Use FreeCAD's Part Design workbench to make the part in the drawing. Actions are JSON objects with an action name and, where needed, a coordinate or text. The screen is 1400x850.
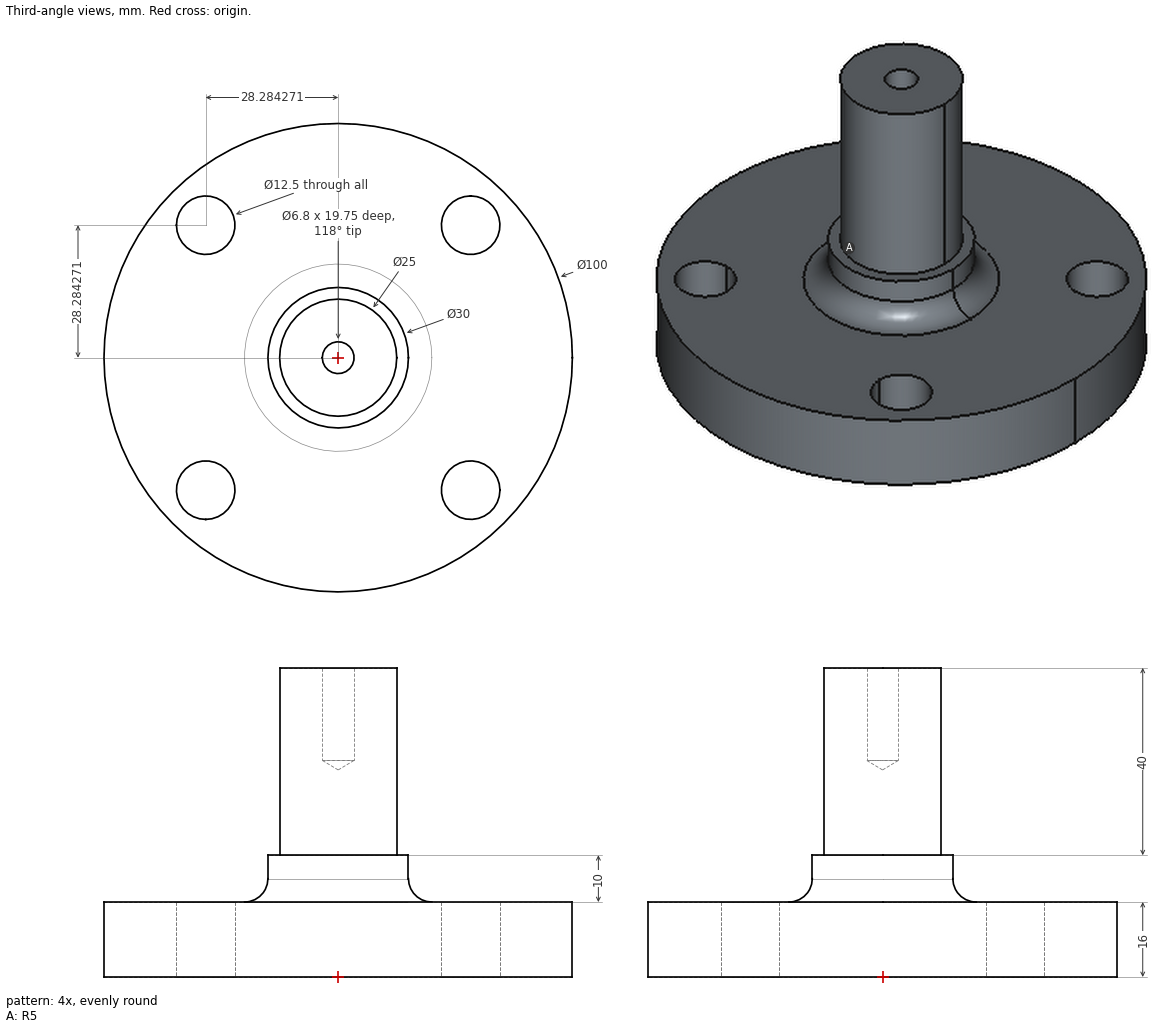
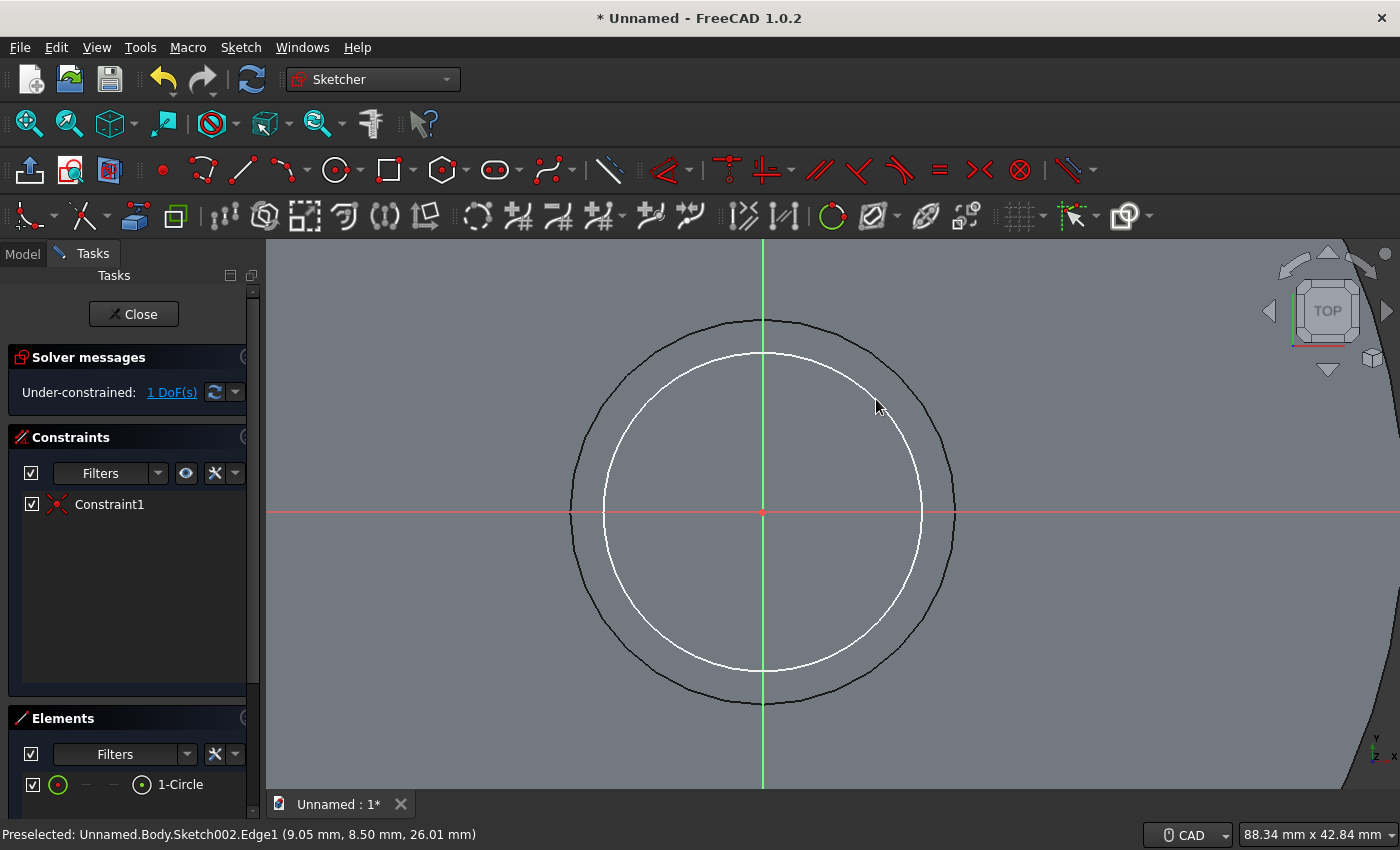
{"action": "left_click", "coordinate": [664, 170]}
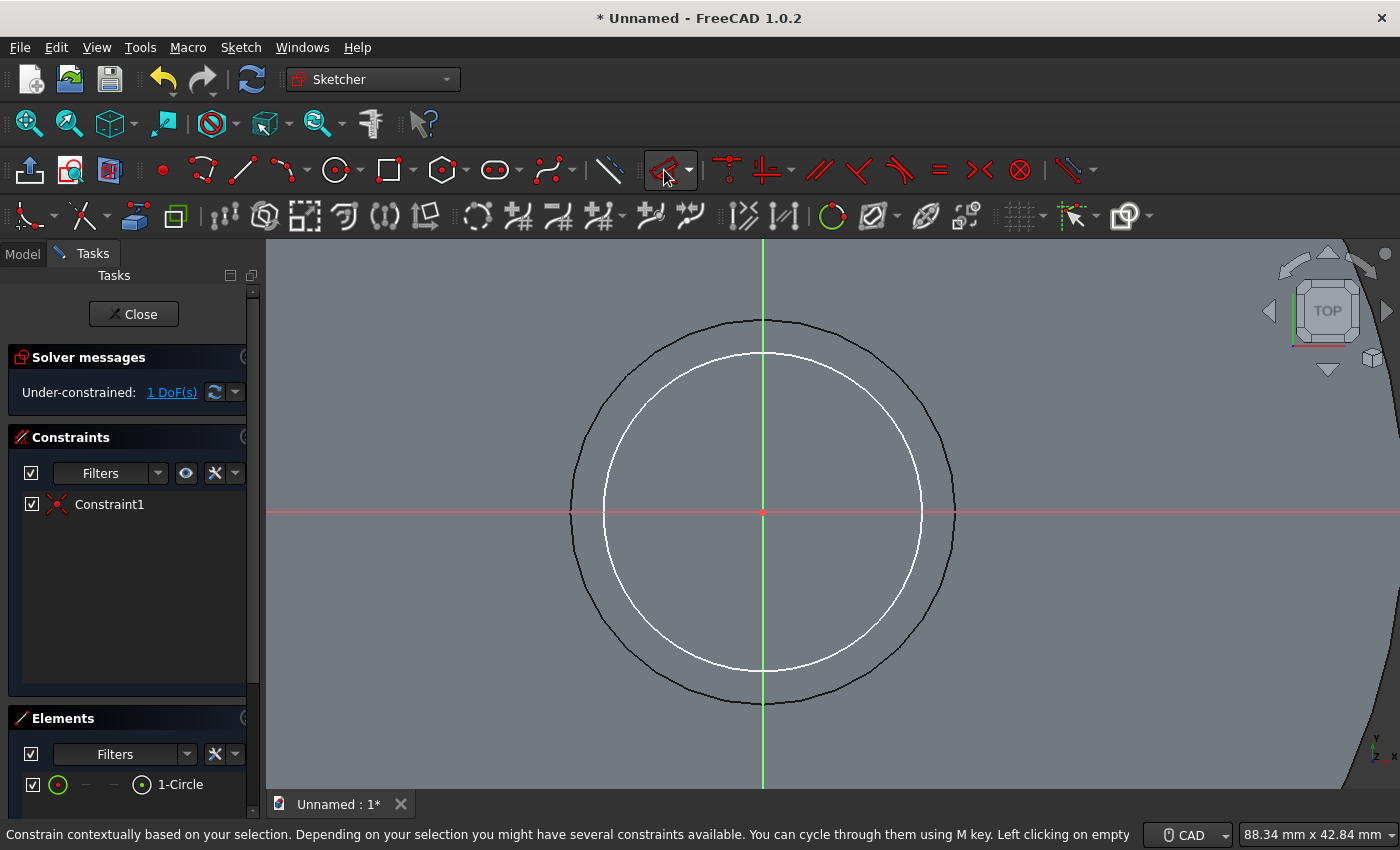
{"action": "left_click", "coordinate": [875, 399]}
{"action": "left_click", "coordinate": [898, 376]}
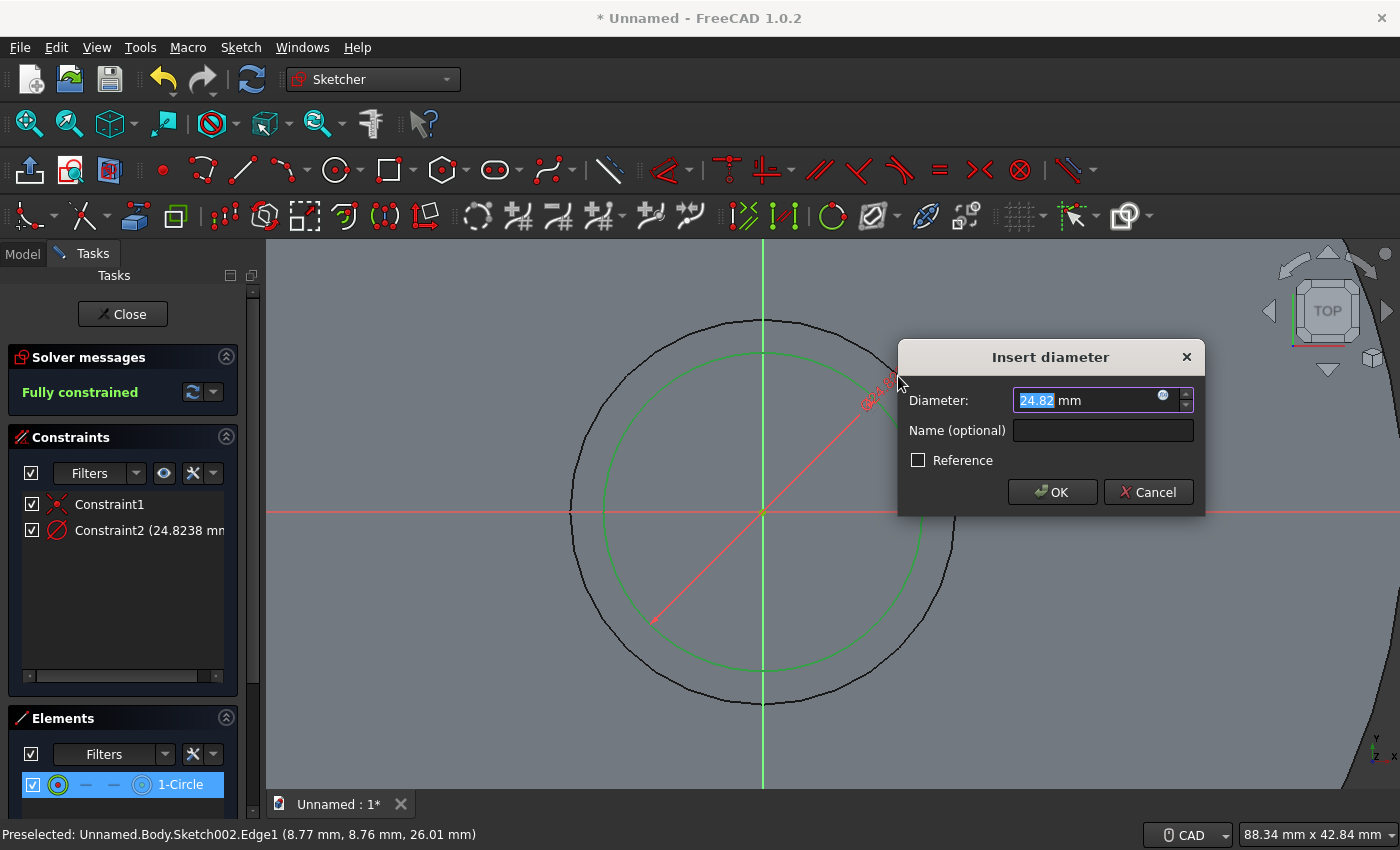
{"action": "type", "text": "25"}
{"action": "key", "text": "Return"}
{"action": "key", "text": "Escape"}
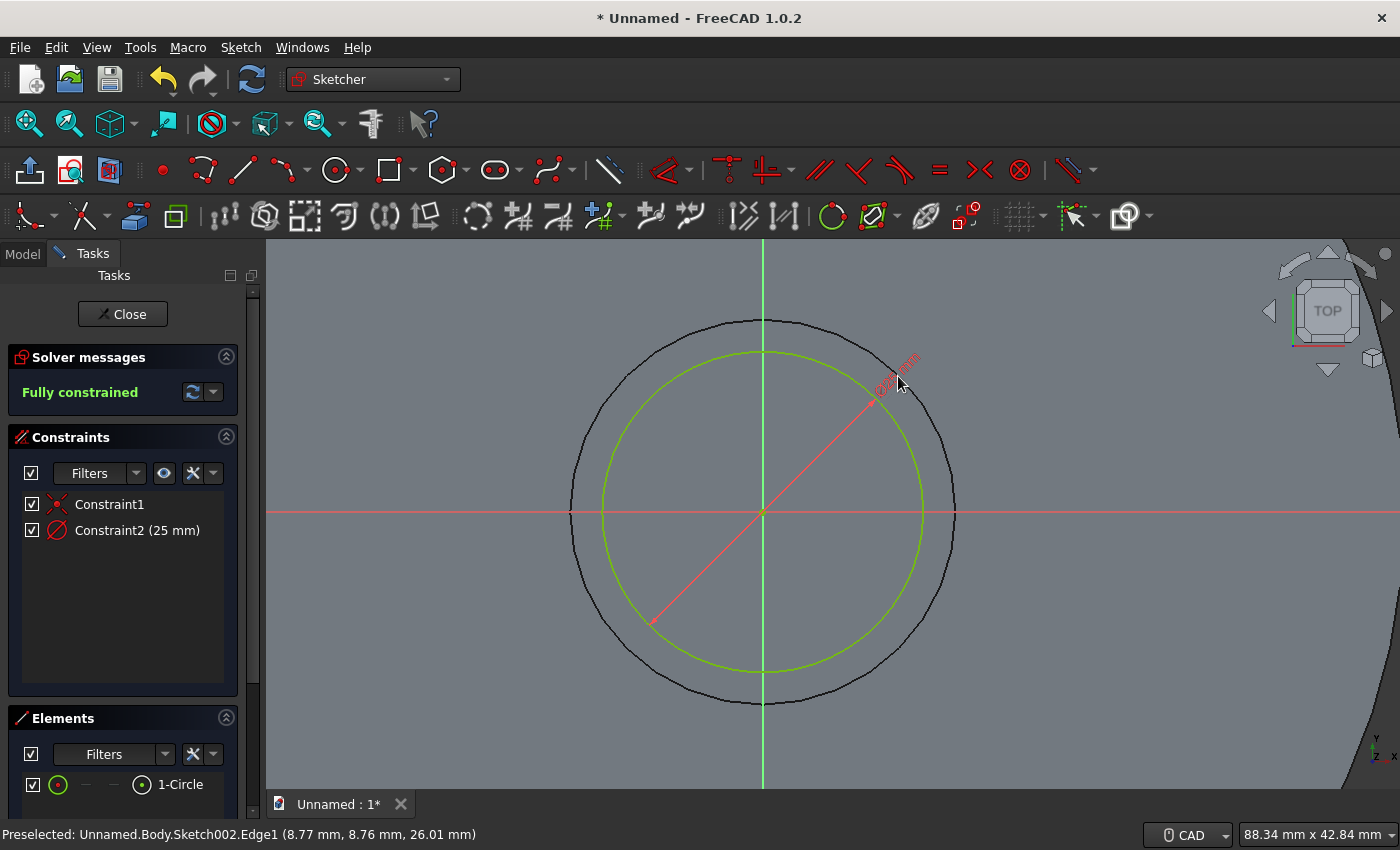
{"action": "left_click", "coordinate": [123, 314]}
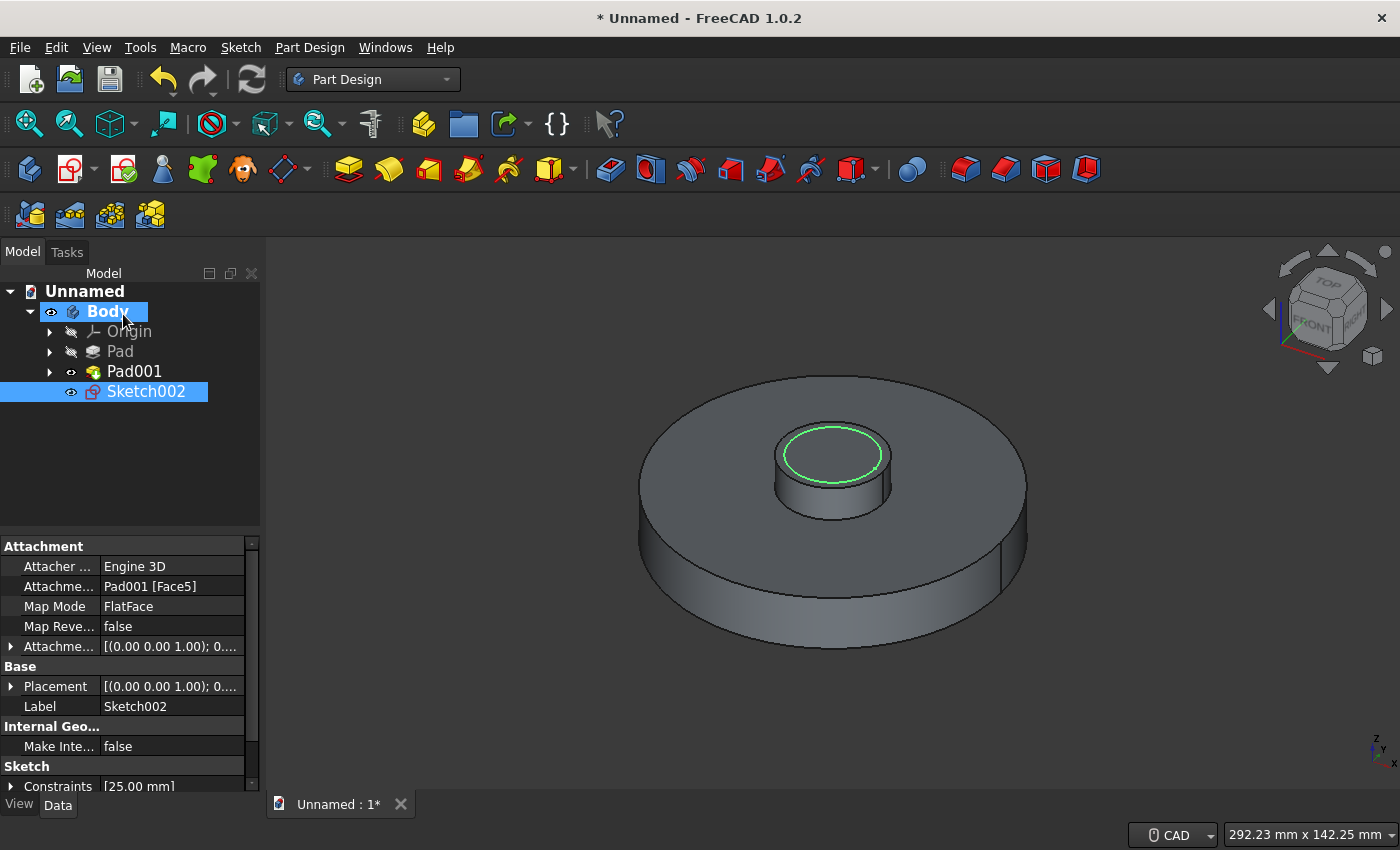
{"action": "left_click", "coordinate": [350, 170]}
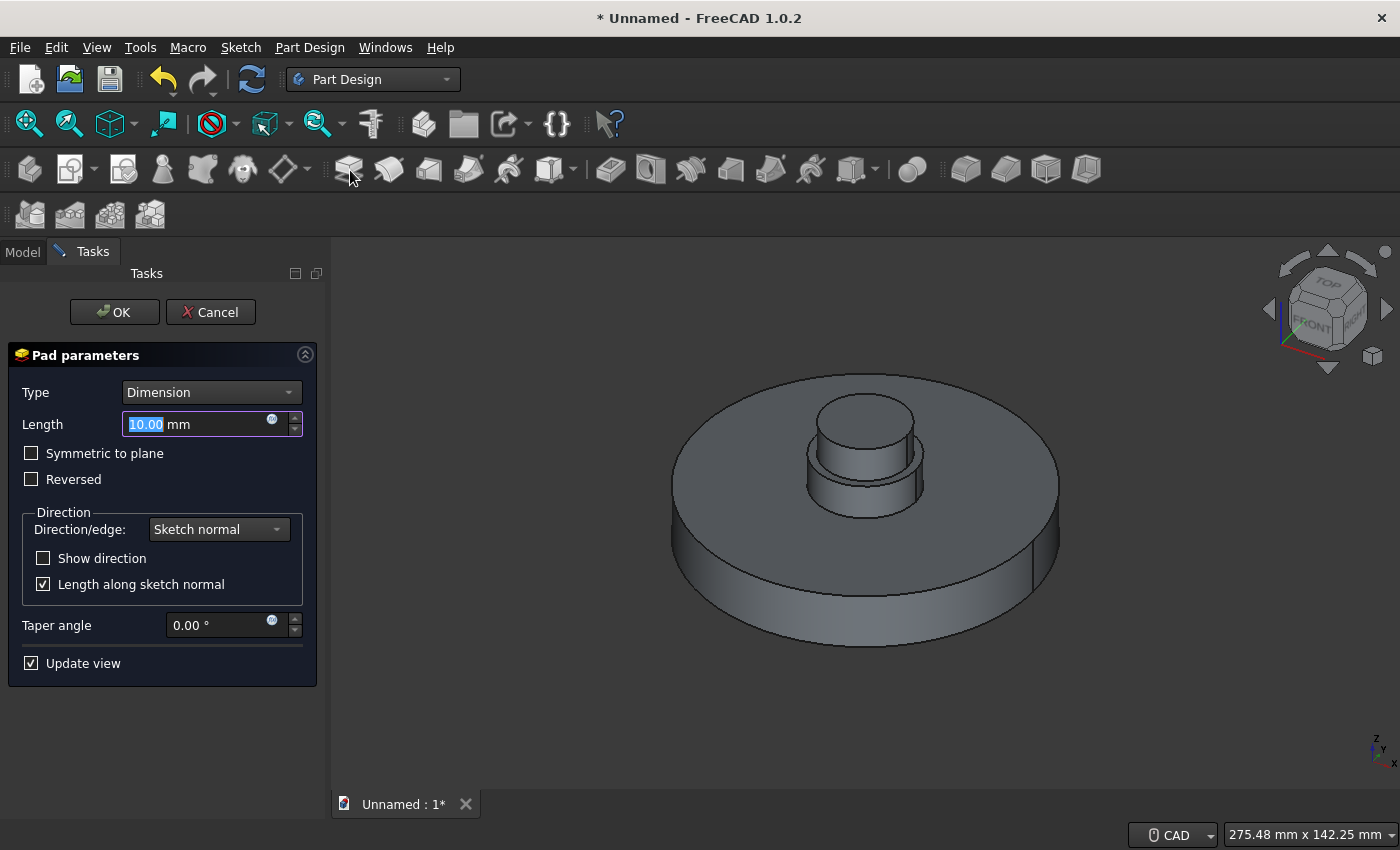
{"action": "type", "text": "40"}
{"action": "key", "text": "Tab"}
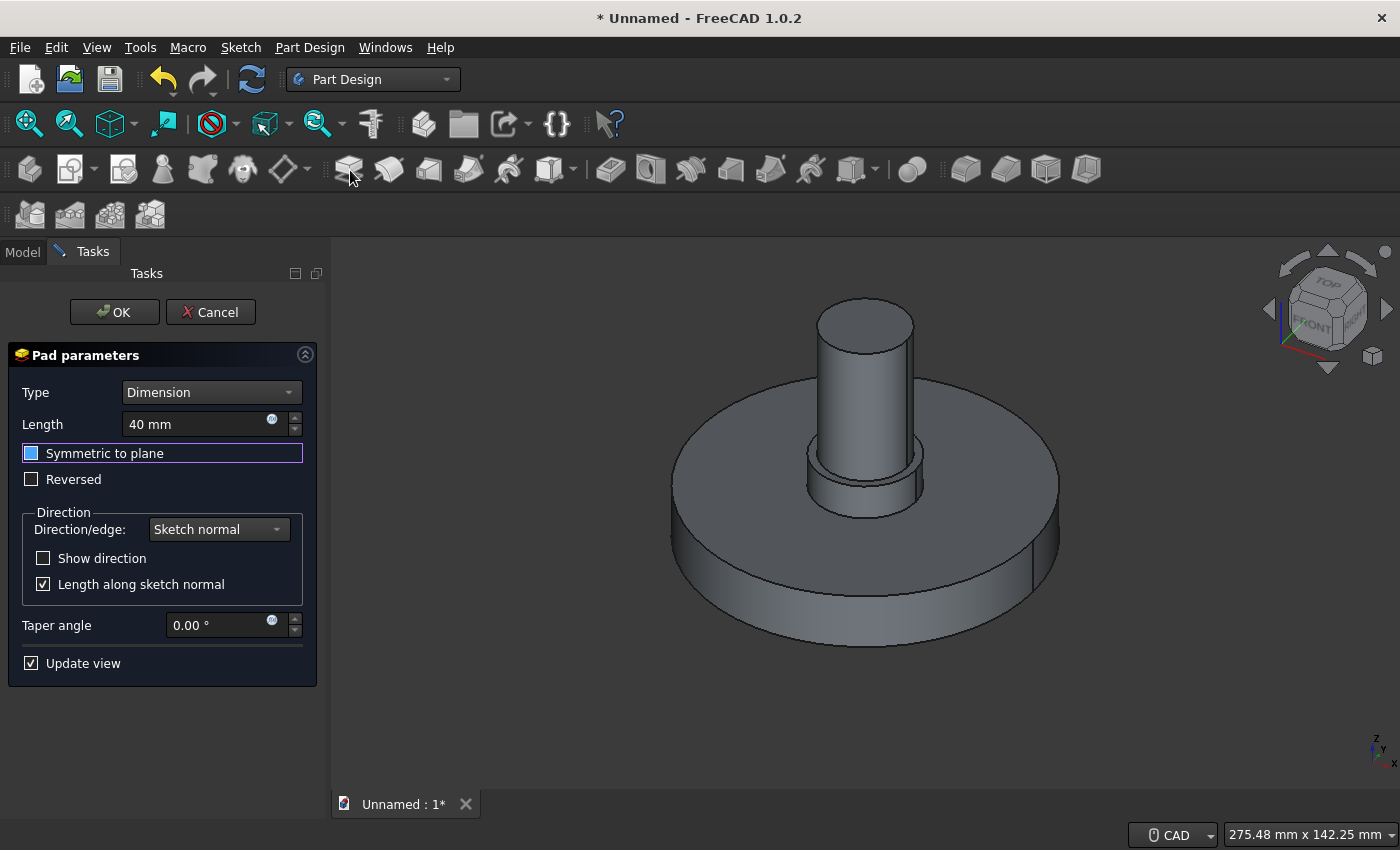
{"action": "left_click", "coordinate": [115, 312]}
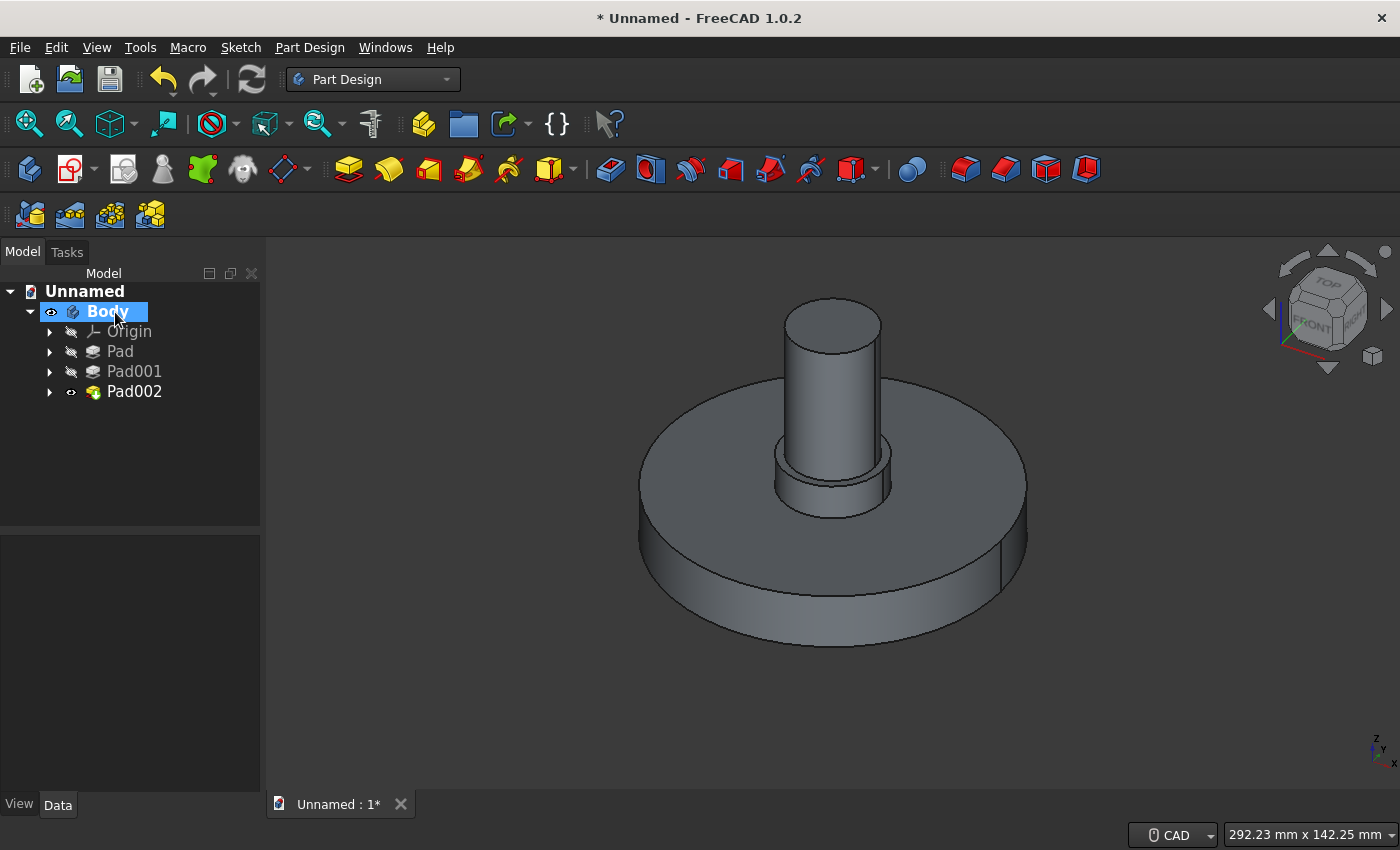
{"action": "left_click", "coordinate": [30, 124]}